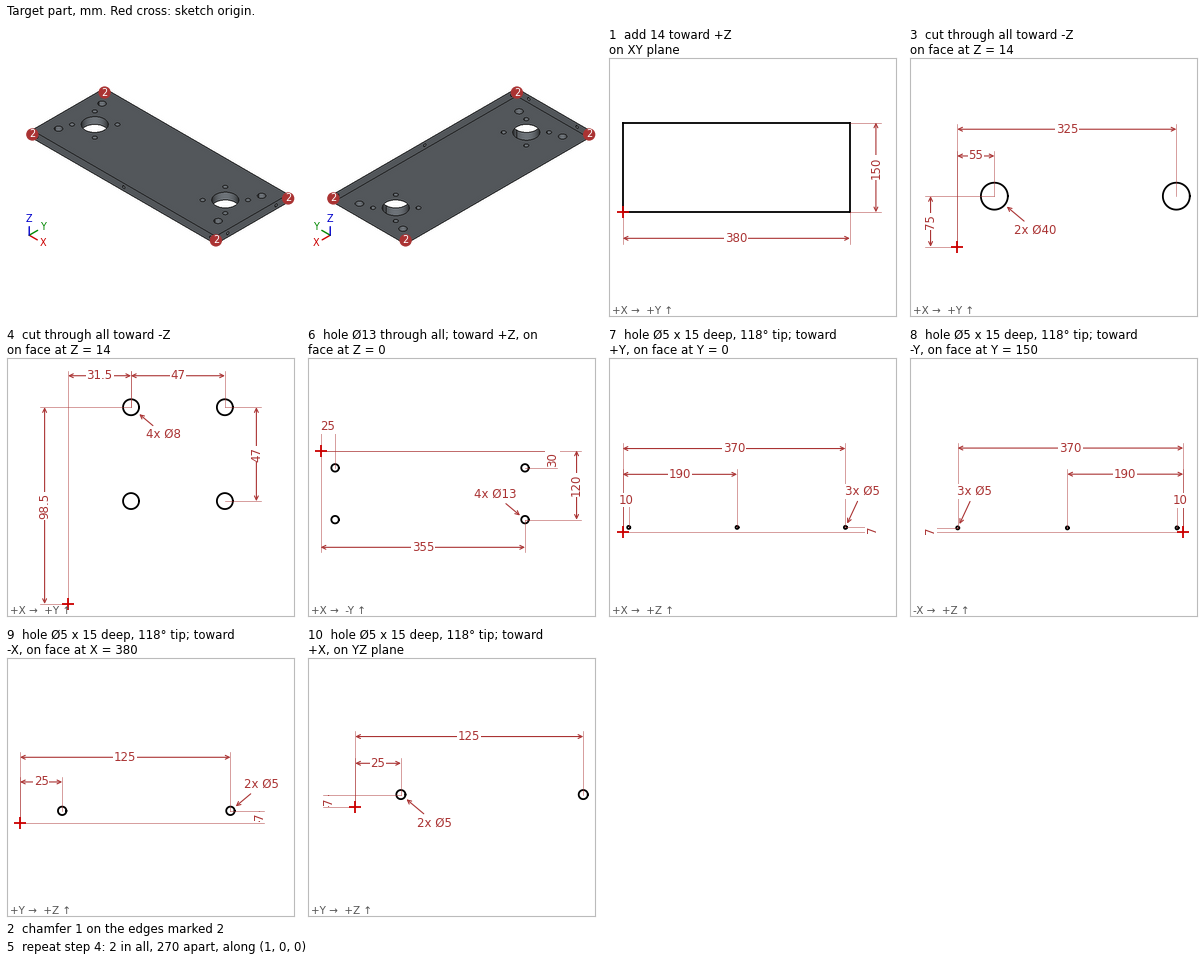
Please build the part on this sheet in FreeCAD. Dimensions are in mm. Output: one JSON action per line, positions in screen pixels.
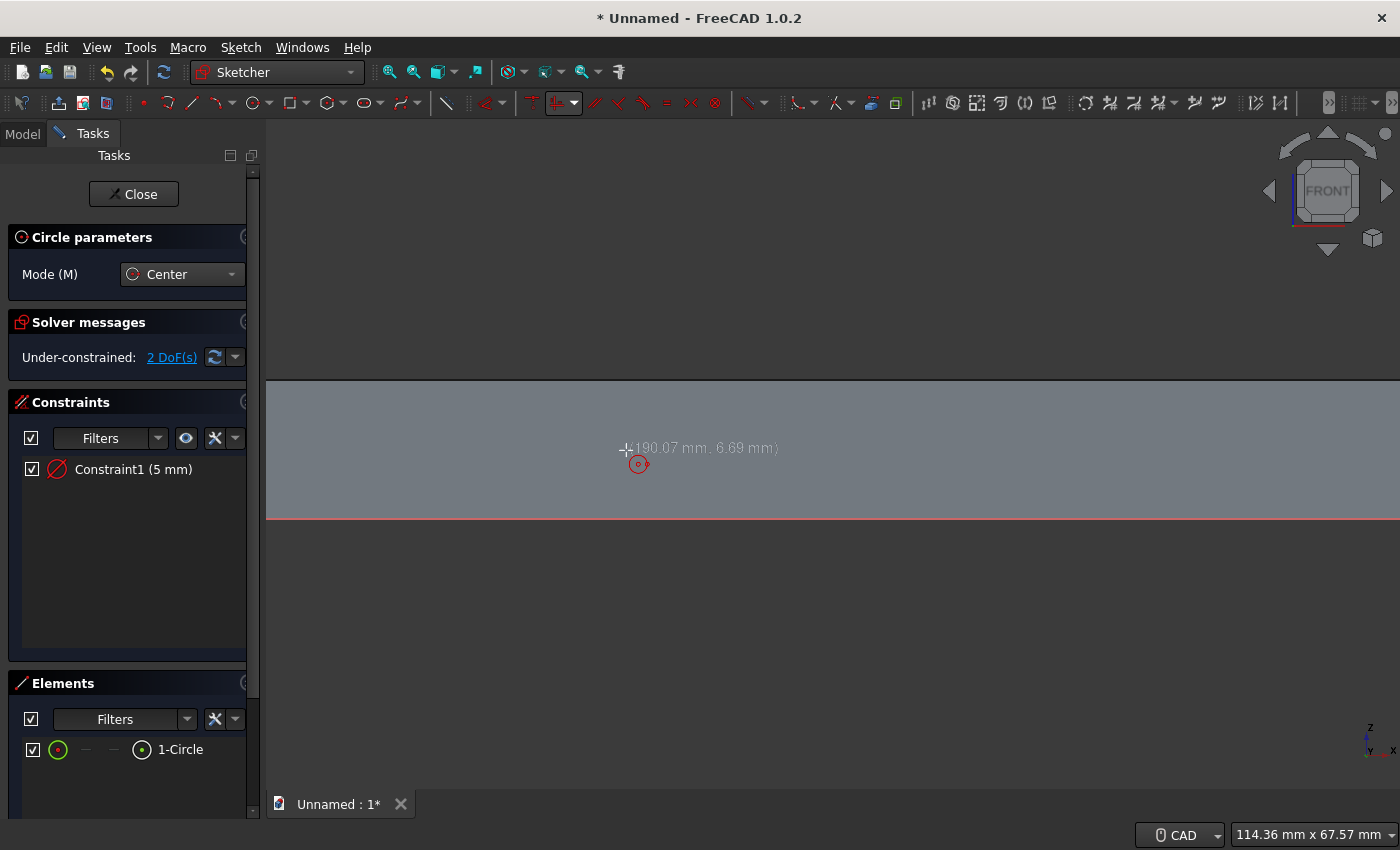
{"action": "scroll", "coordinate": [800, 450], "scroll_direction": "down", "scroll_amount": 9}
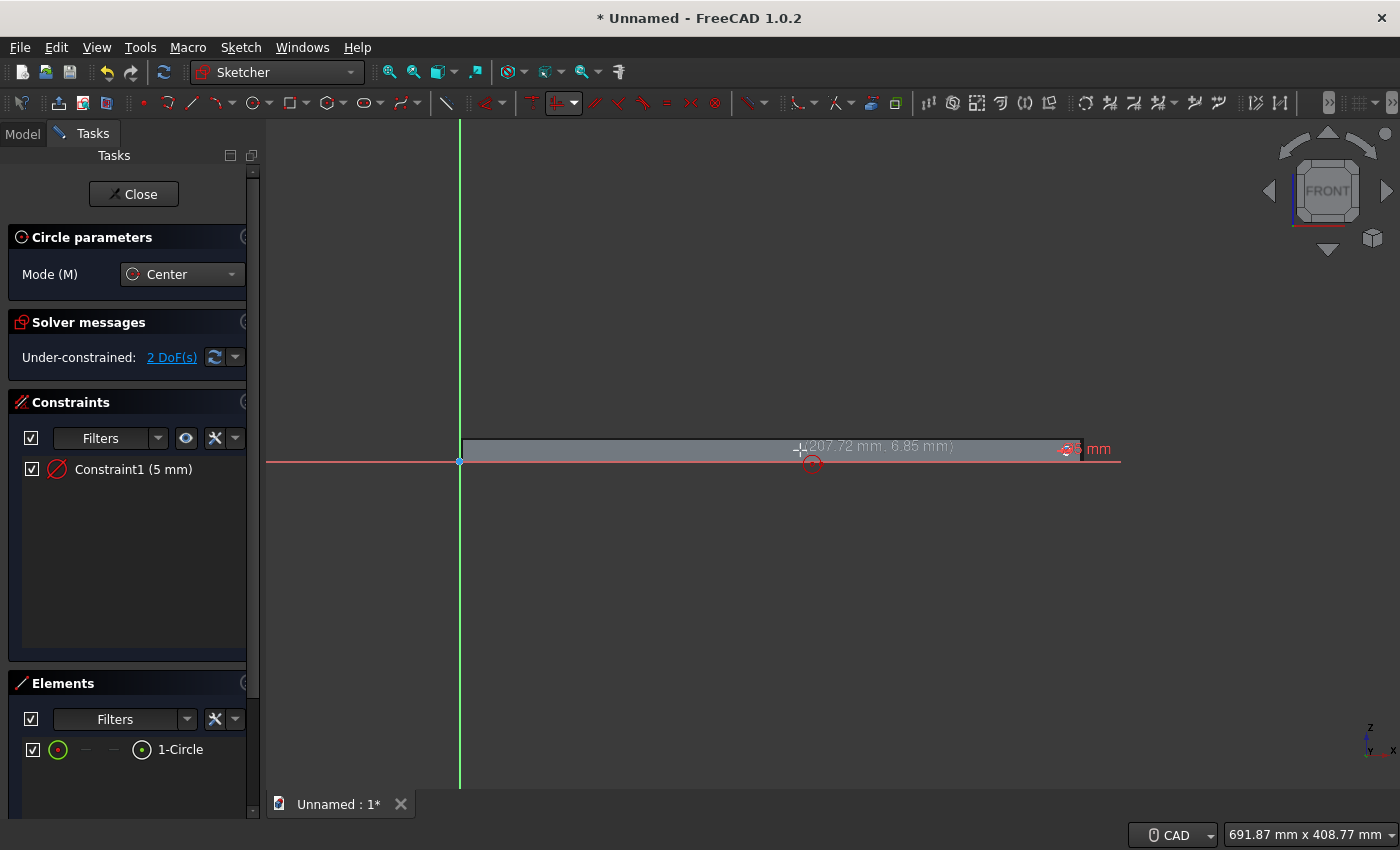
{"action": "scroll", "coordinate": [771, 450], "scroll_direction": "up", "scroll_amount": 2}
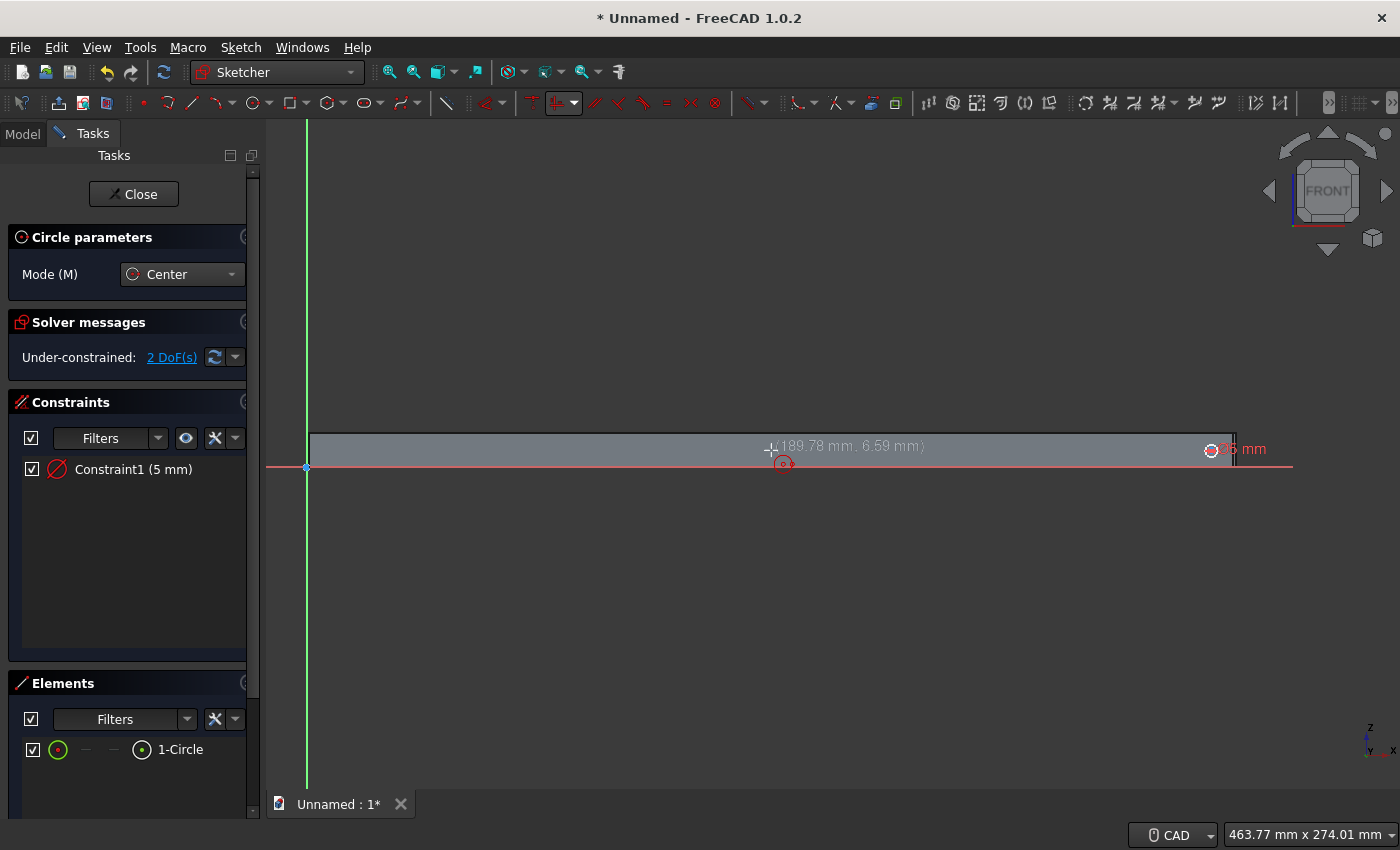
{"action": "left_click", "coordinate": [771, 450]}
{"action": "mouse_move", "coordinate": [776, 446]}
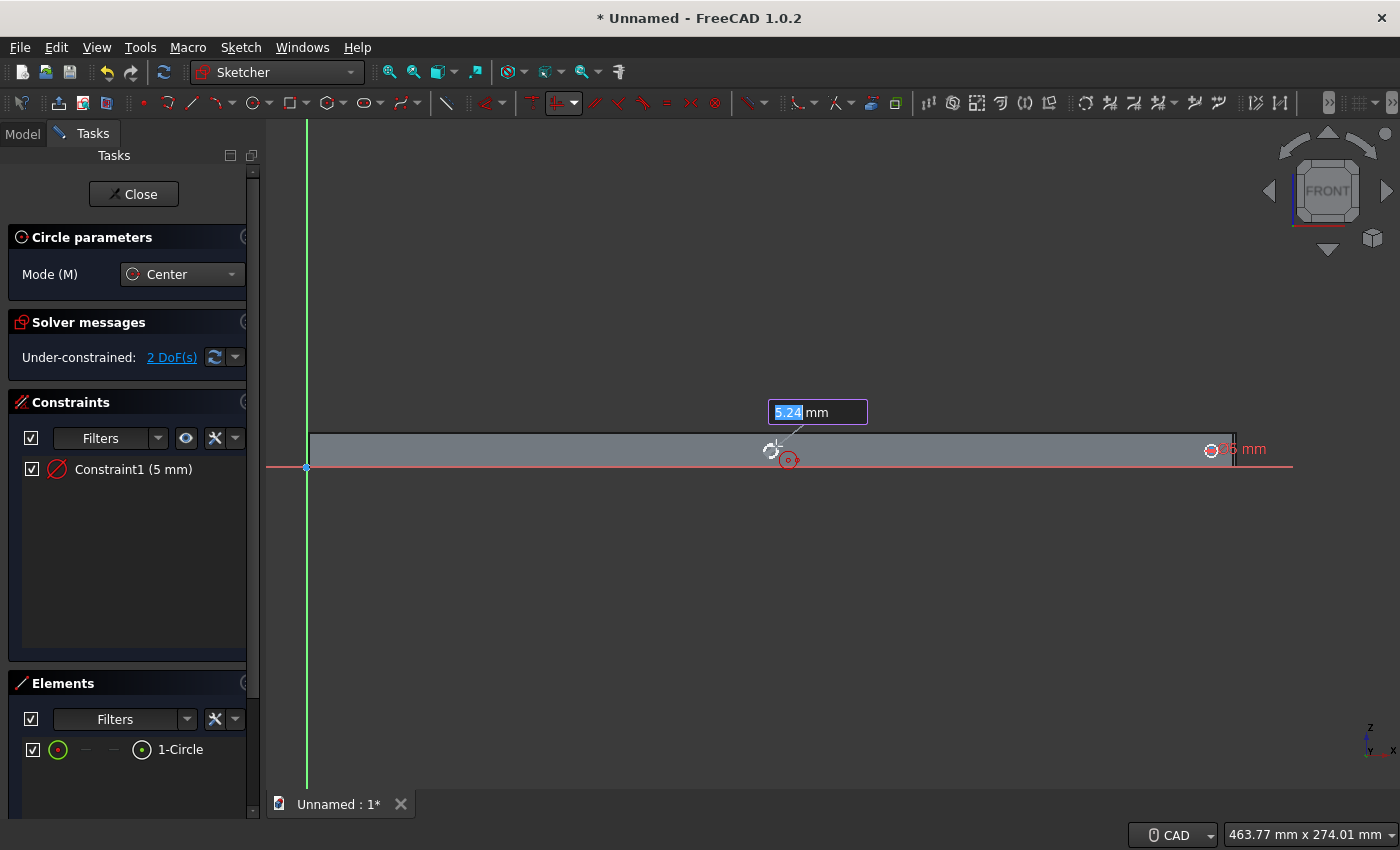
{"action": "type", "text": "5"}
{"action": "key", "text": "Return"}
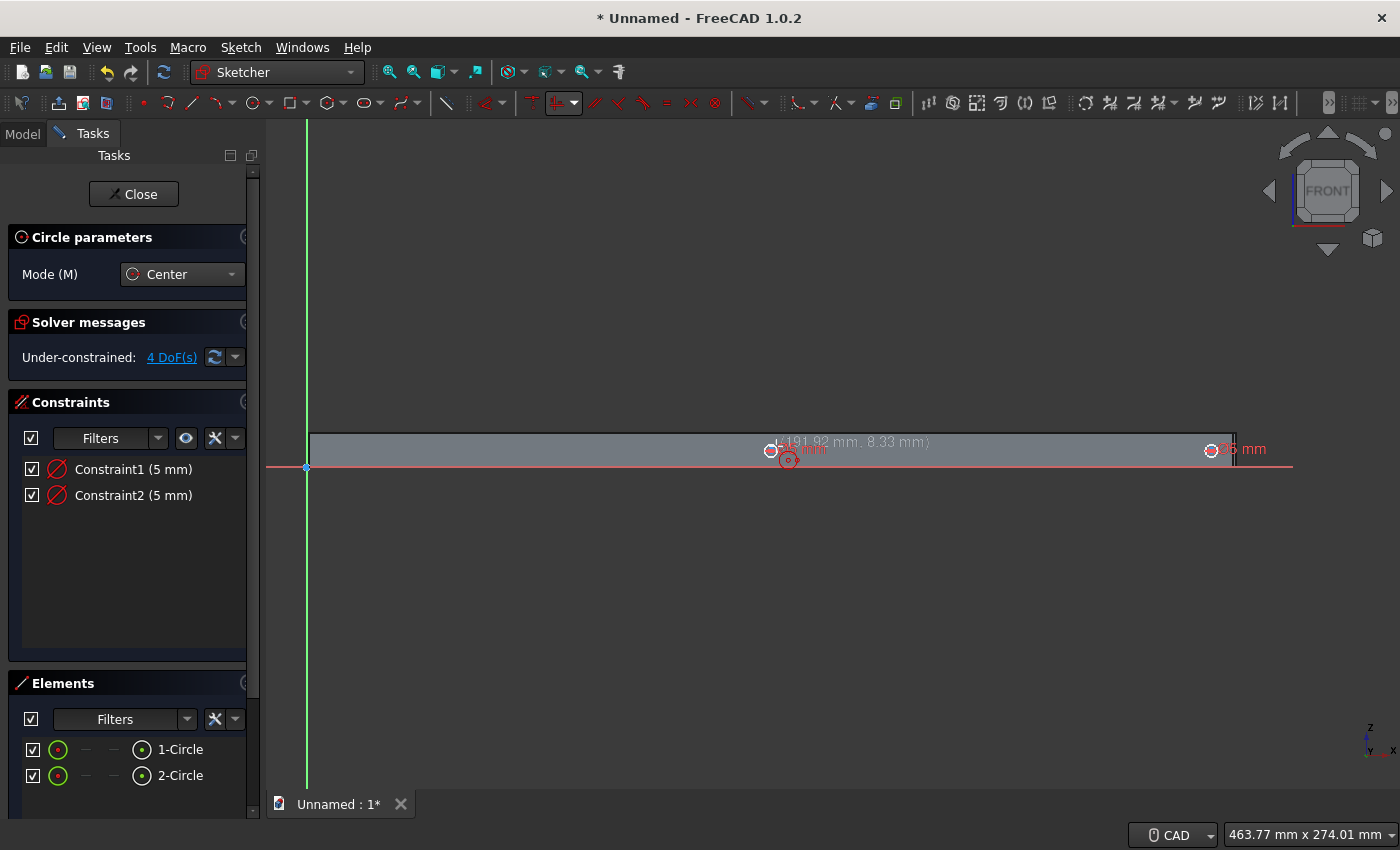
{"action": "scroll", "coordinate": [331, 450], "scroll_direction": "up", "scroll_amount": 7}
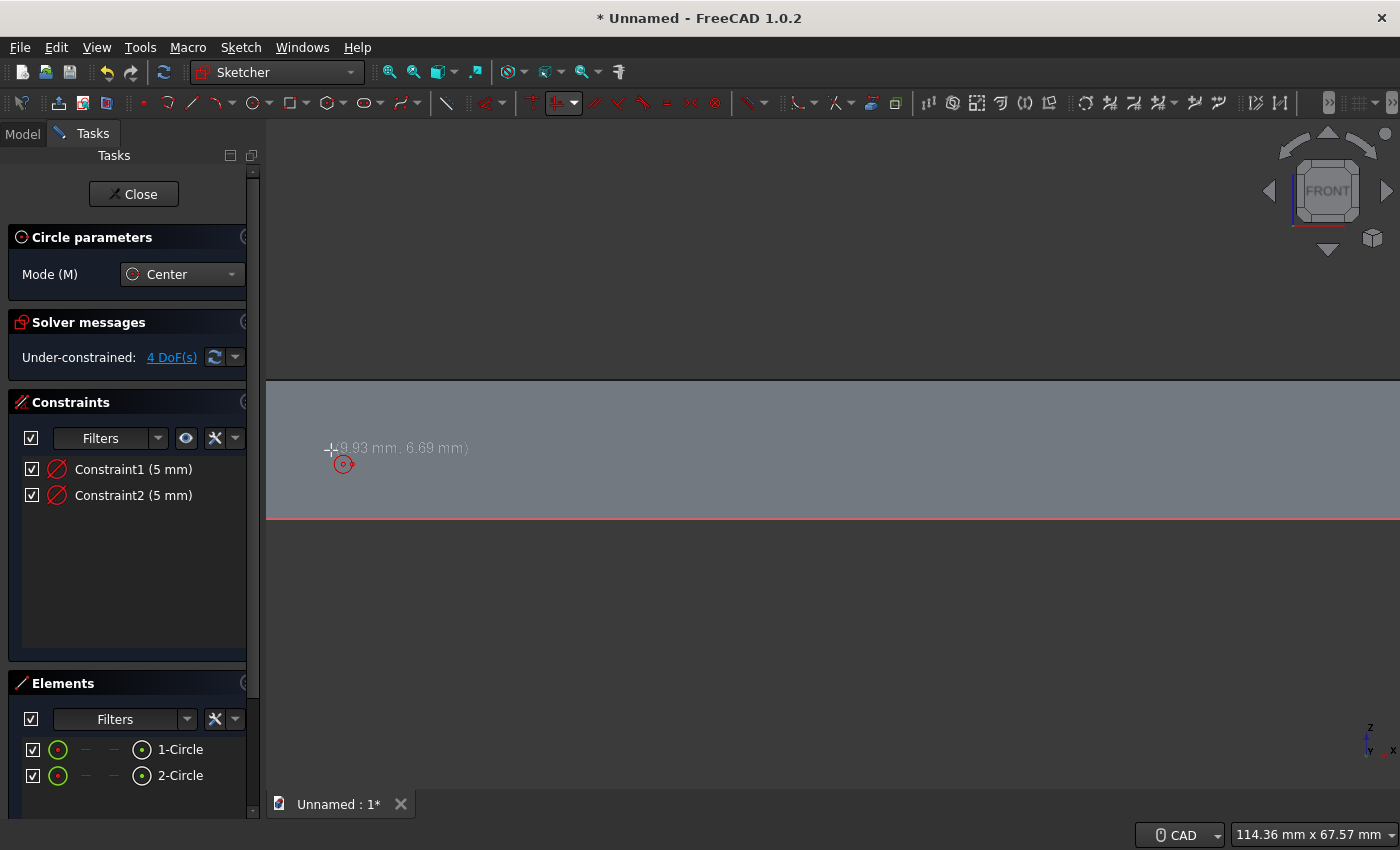
{"action": "scroll", "coordinate": [504, 450], "scroll_direction": "down", "scroll_amount": 9}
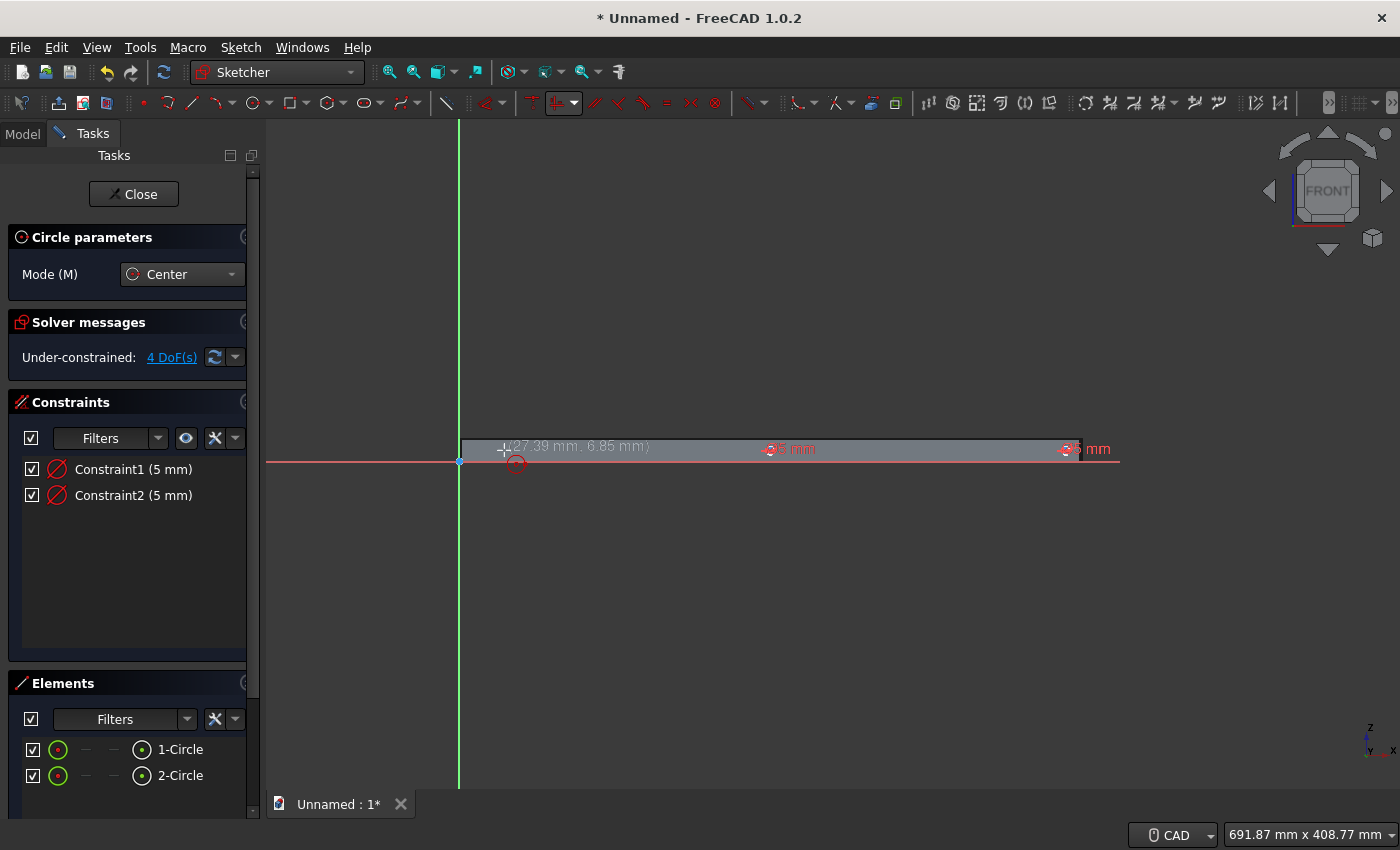
{"action": "scroll", "coordinate": [476, 450], "scroll_direction": "up", "scroll_amount": 2}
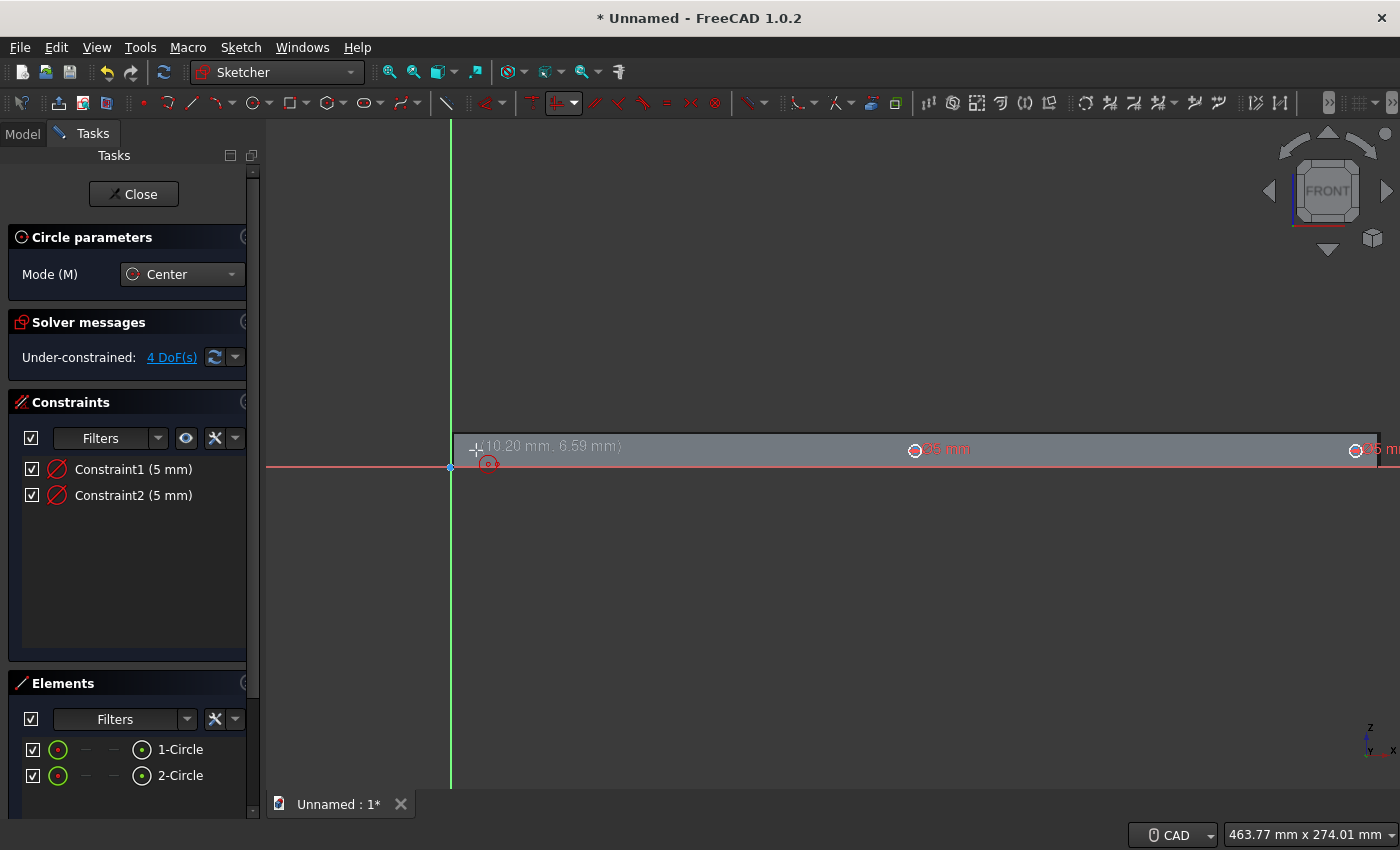
{"action": "left_click", "coordinate": [475, 450]}
{"action": "mouse_move", "coordinate": [480, 446]}